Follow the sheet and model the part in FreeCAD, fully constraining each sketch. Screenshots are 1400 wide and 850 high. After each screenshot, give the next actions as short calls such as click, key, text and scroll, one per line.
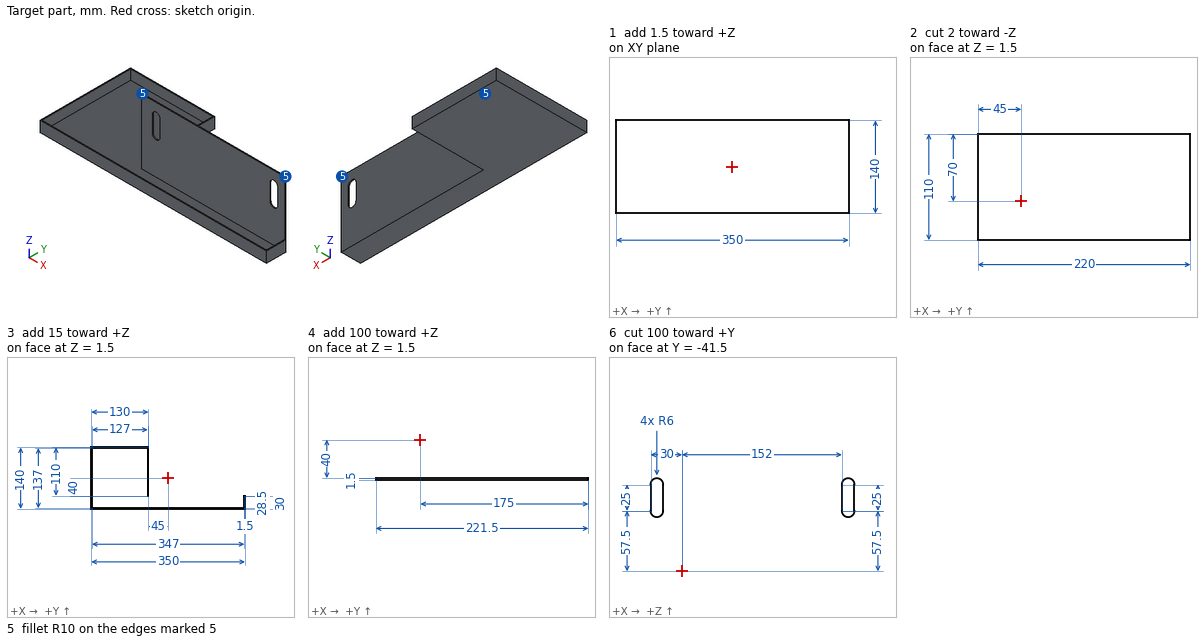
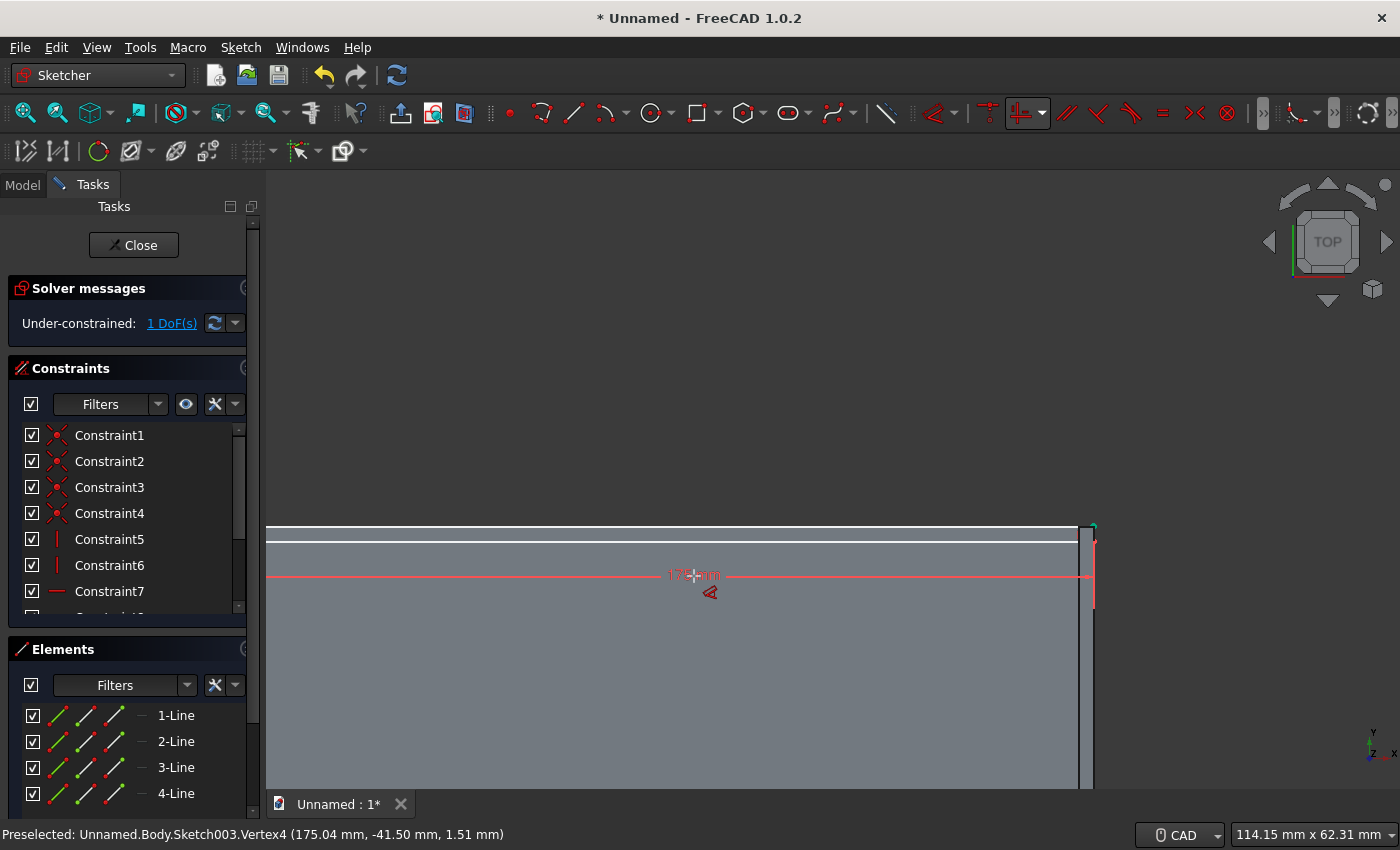
click(434, 542)
click(510, 576)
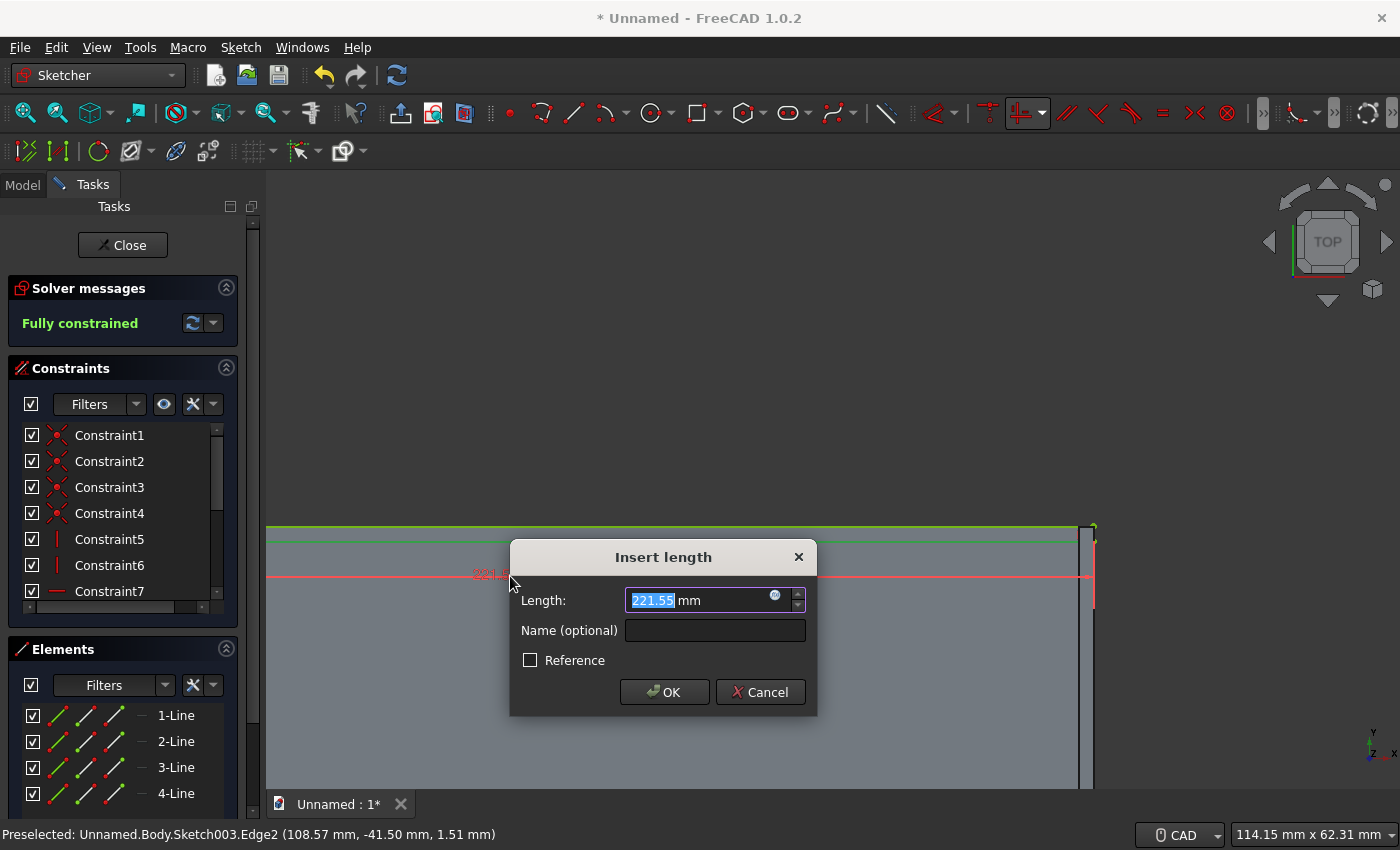
text(221.5)
key(Return)
key(Escape)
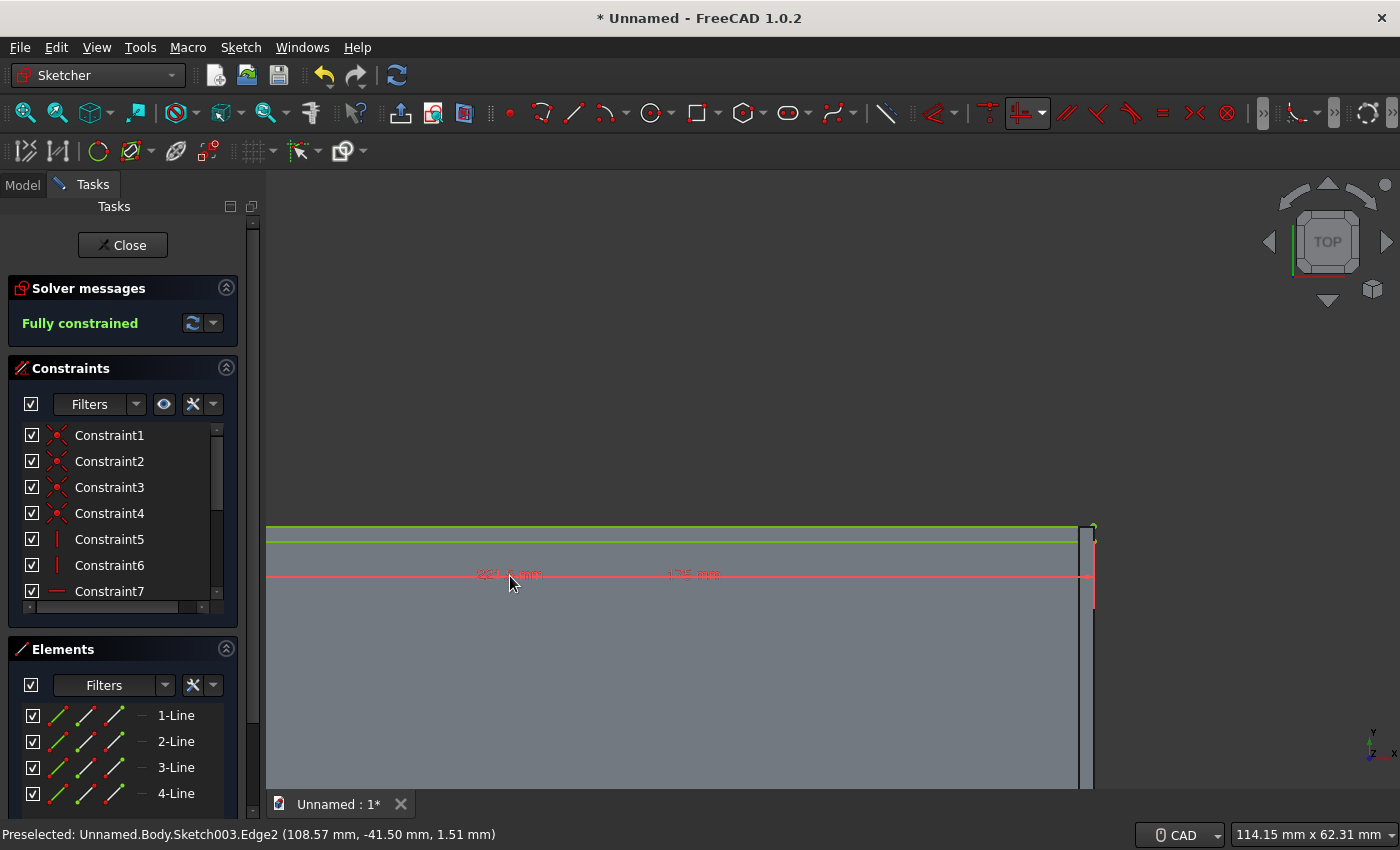
click(123, 245)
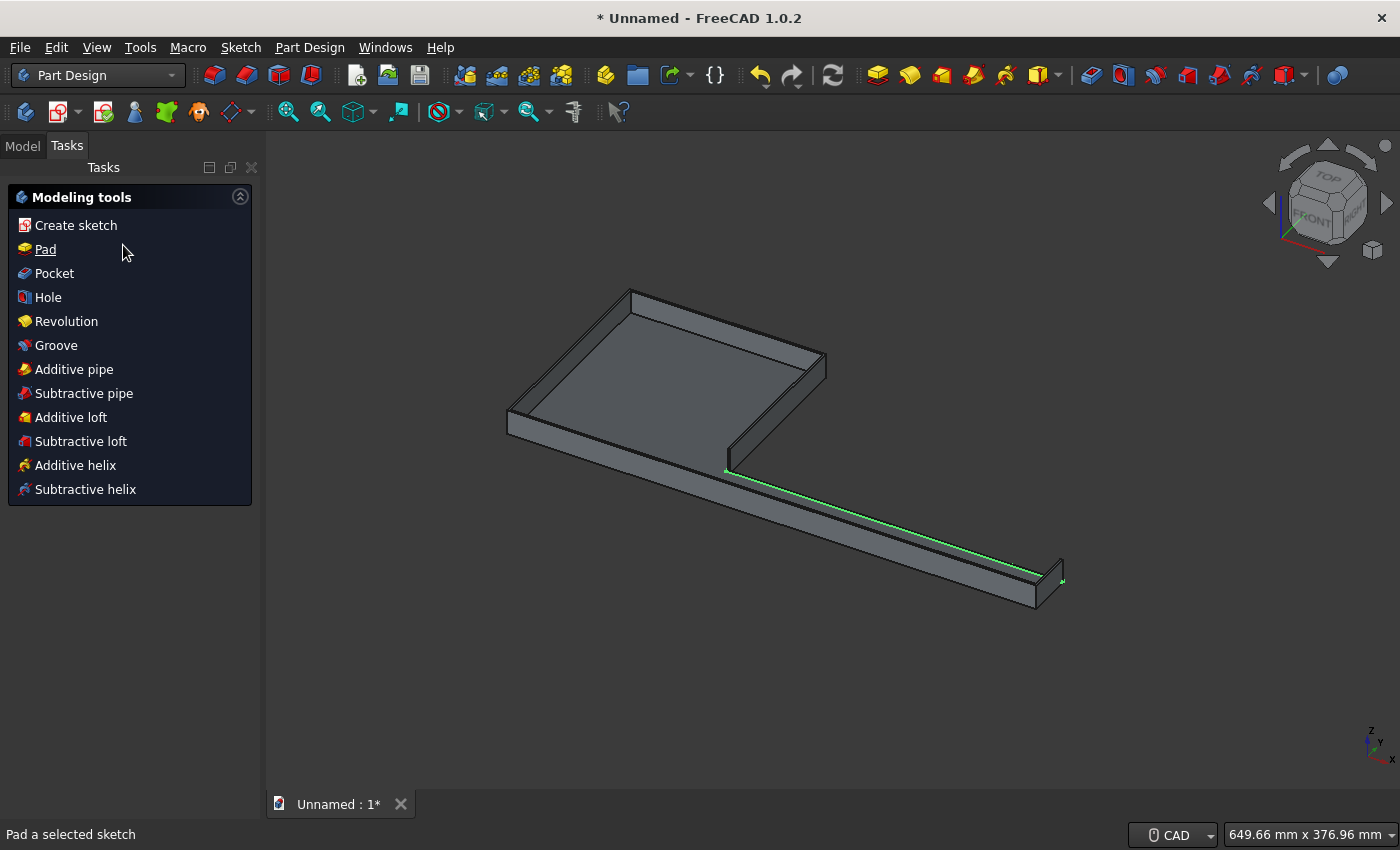
click(878, 76)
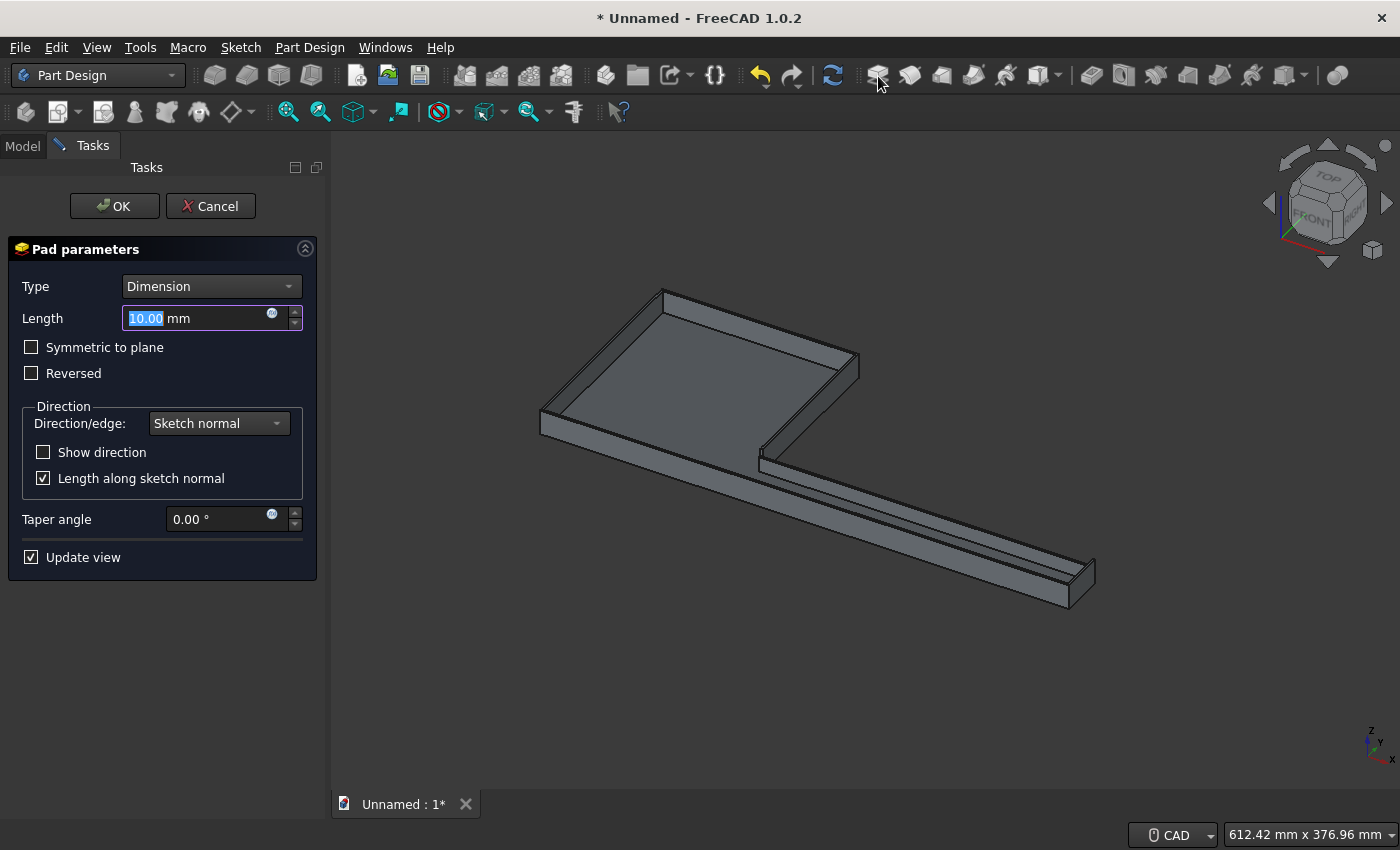
text(100)
key(Tab)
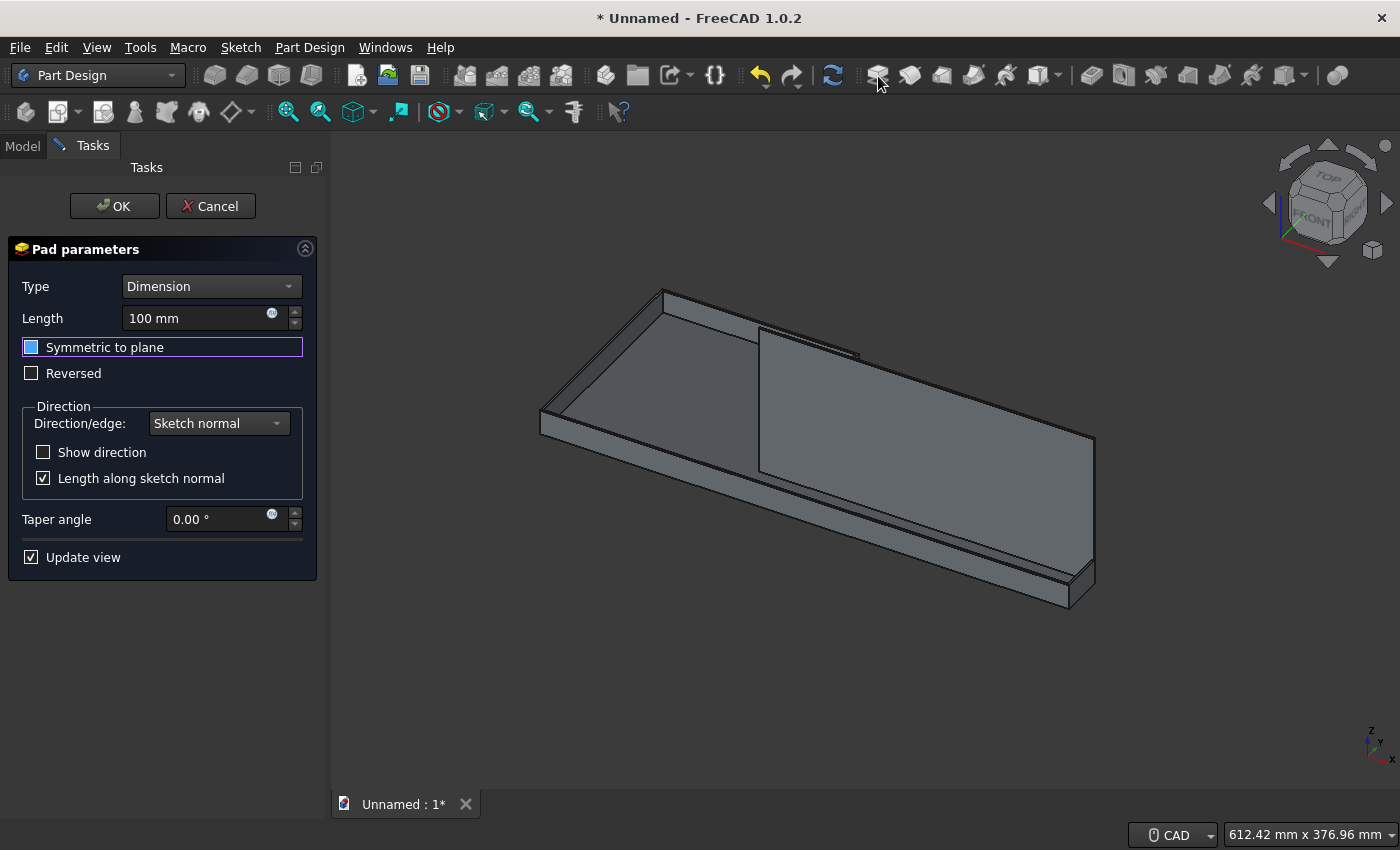
click(115, 206)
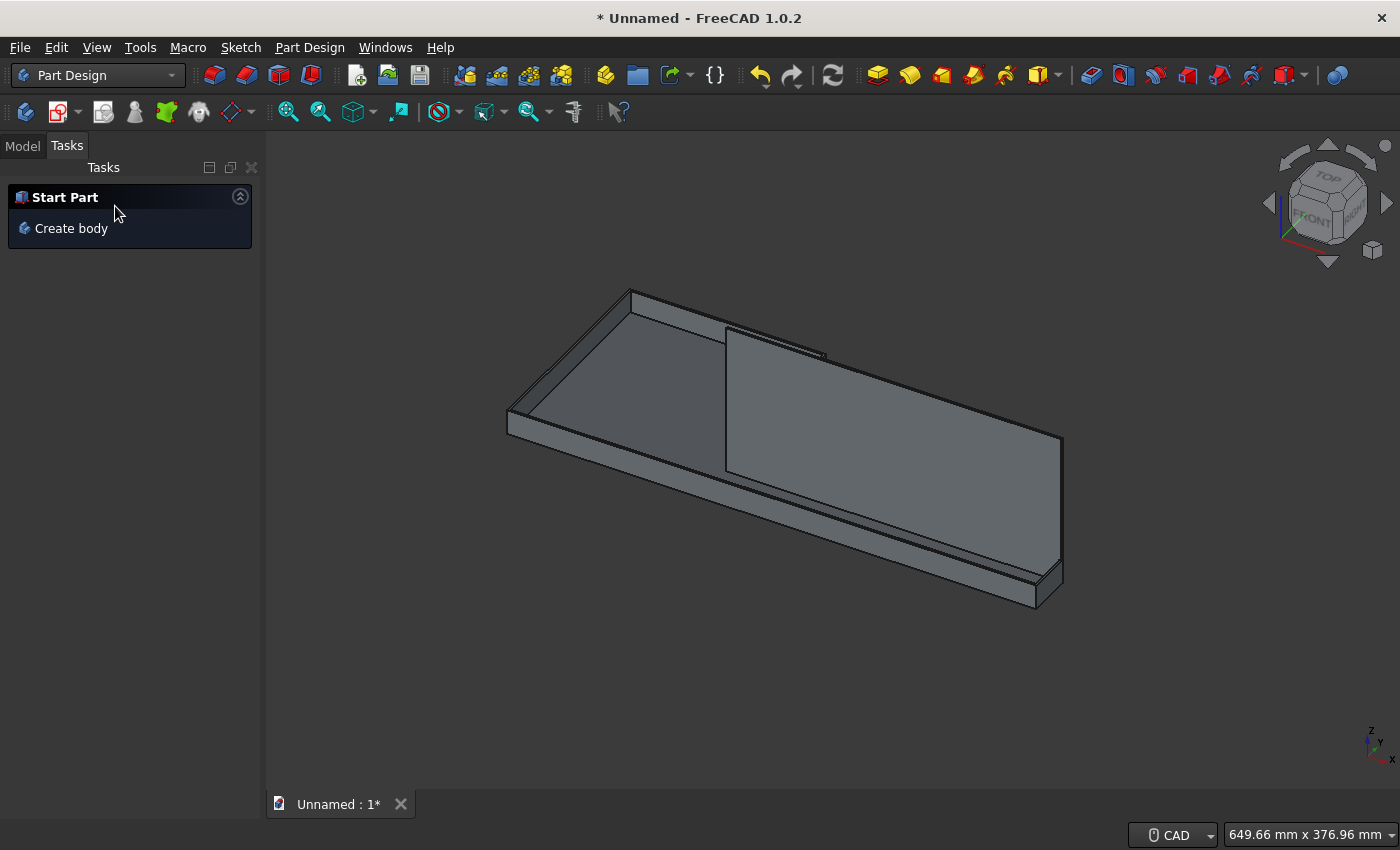
scroll(727, 327, up, 14)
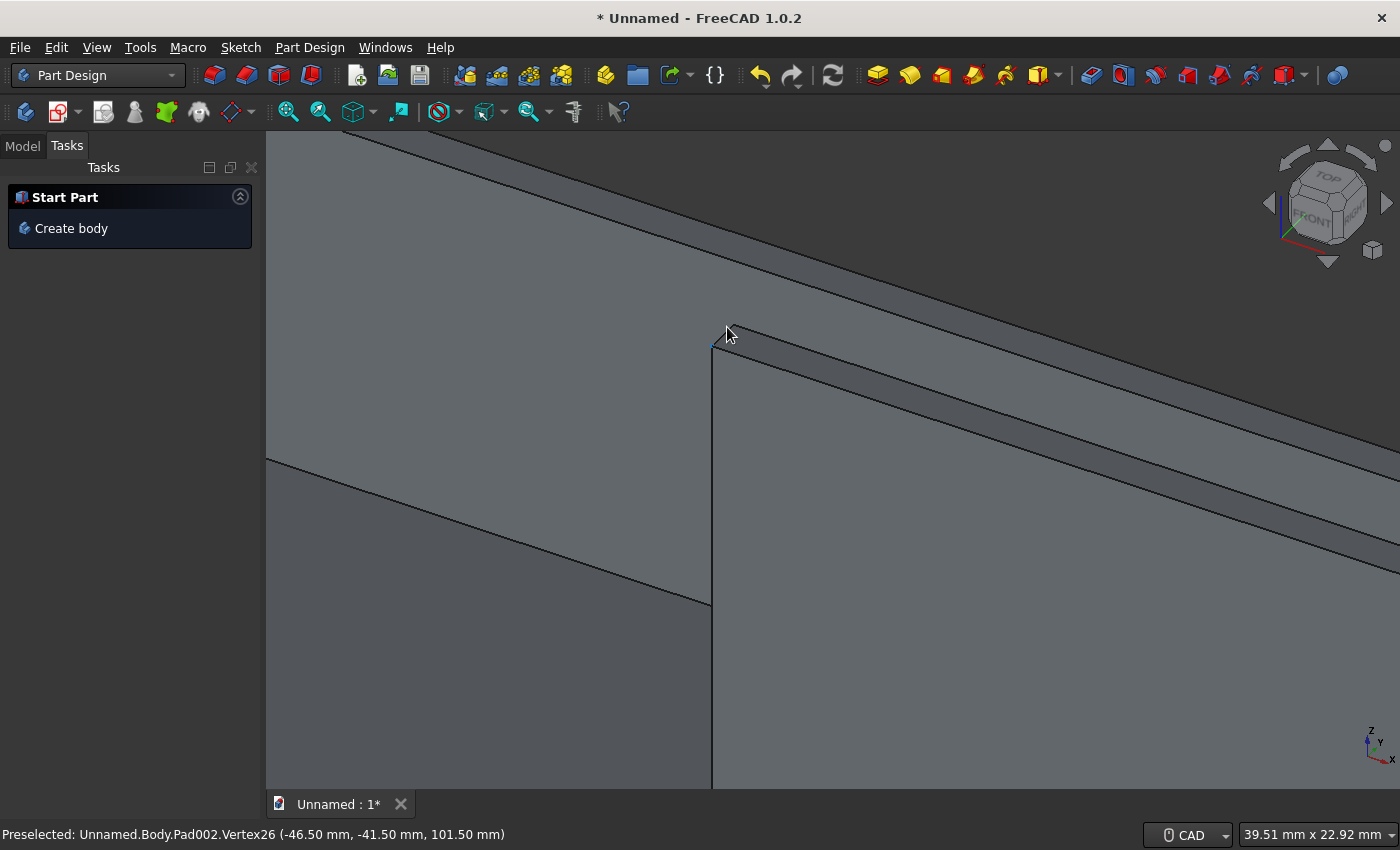
click(290, 112)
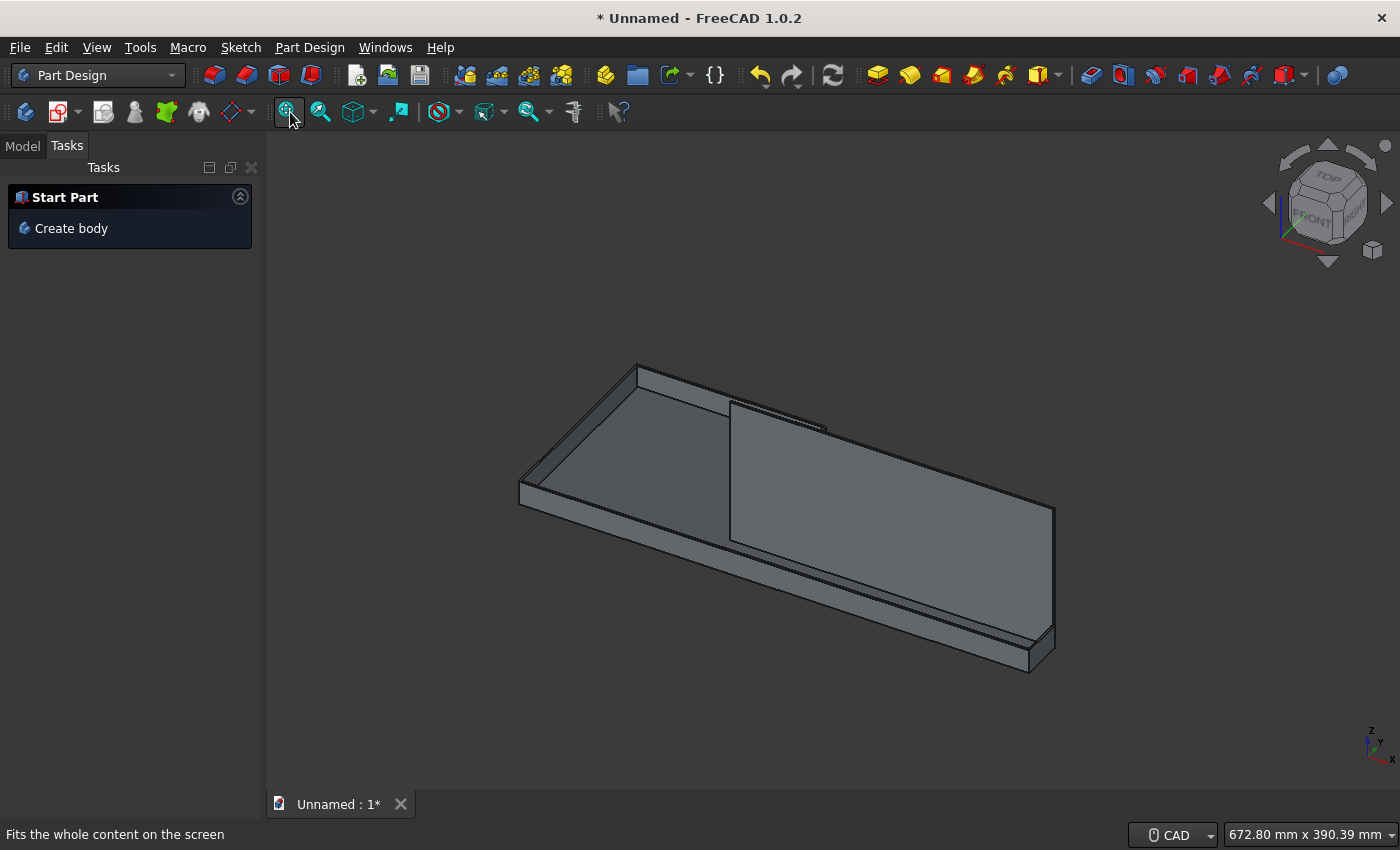
key(0)